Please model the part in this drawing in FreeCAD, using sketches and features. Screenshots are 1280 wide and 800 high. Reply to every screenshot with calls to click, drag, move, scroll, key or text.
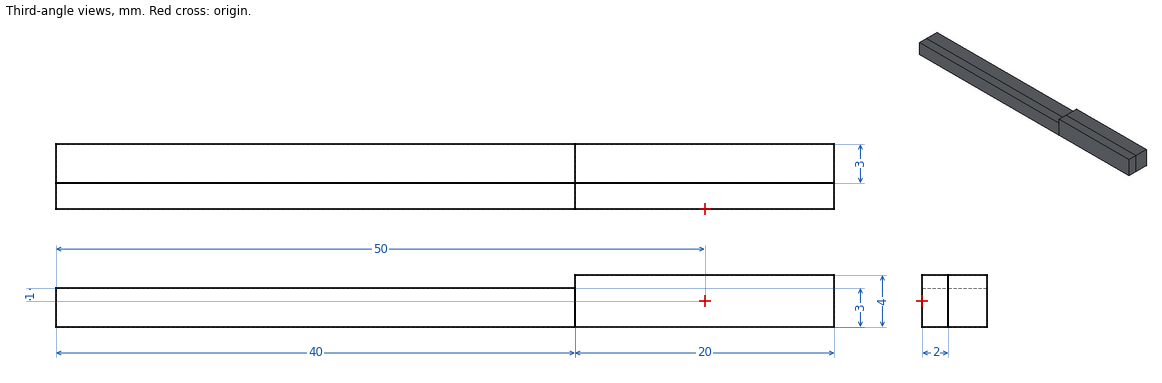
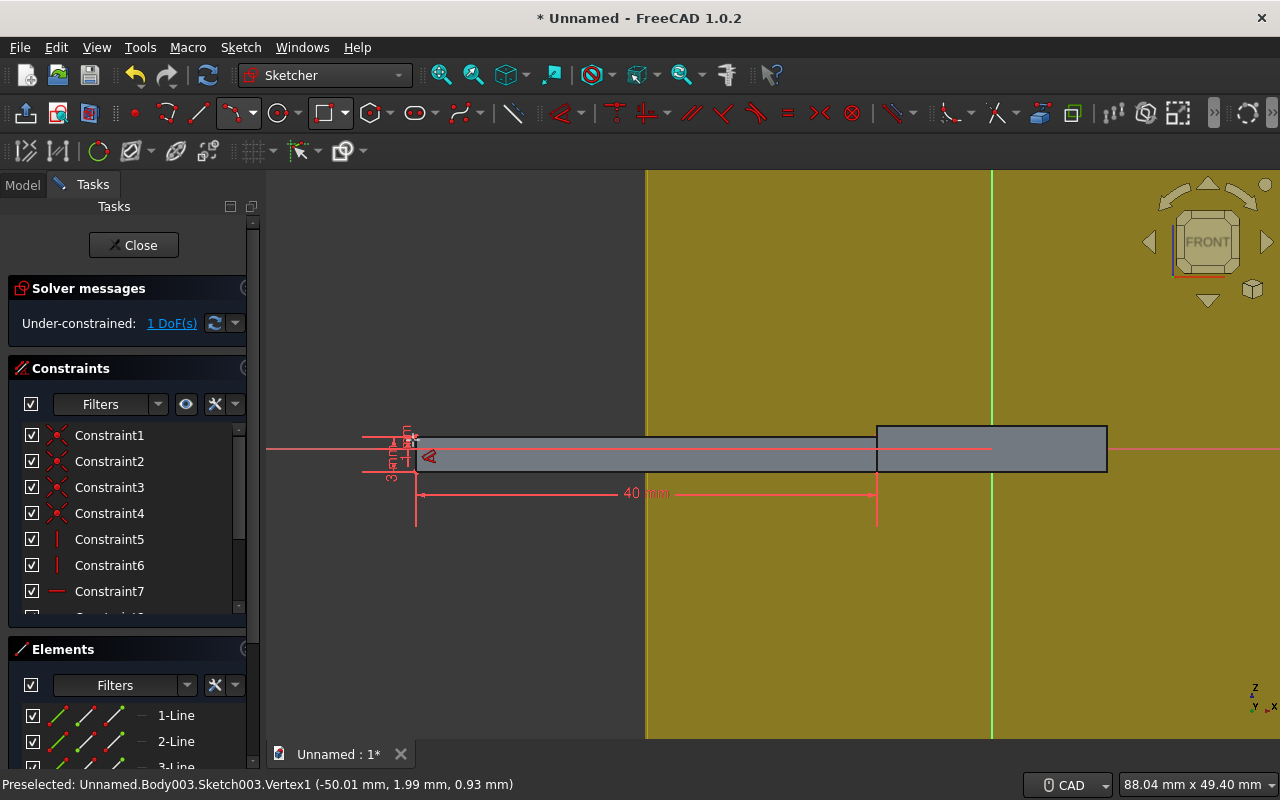
click(416, 437)
click(704, 403)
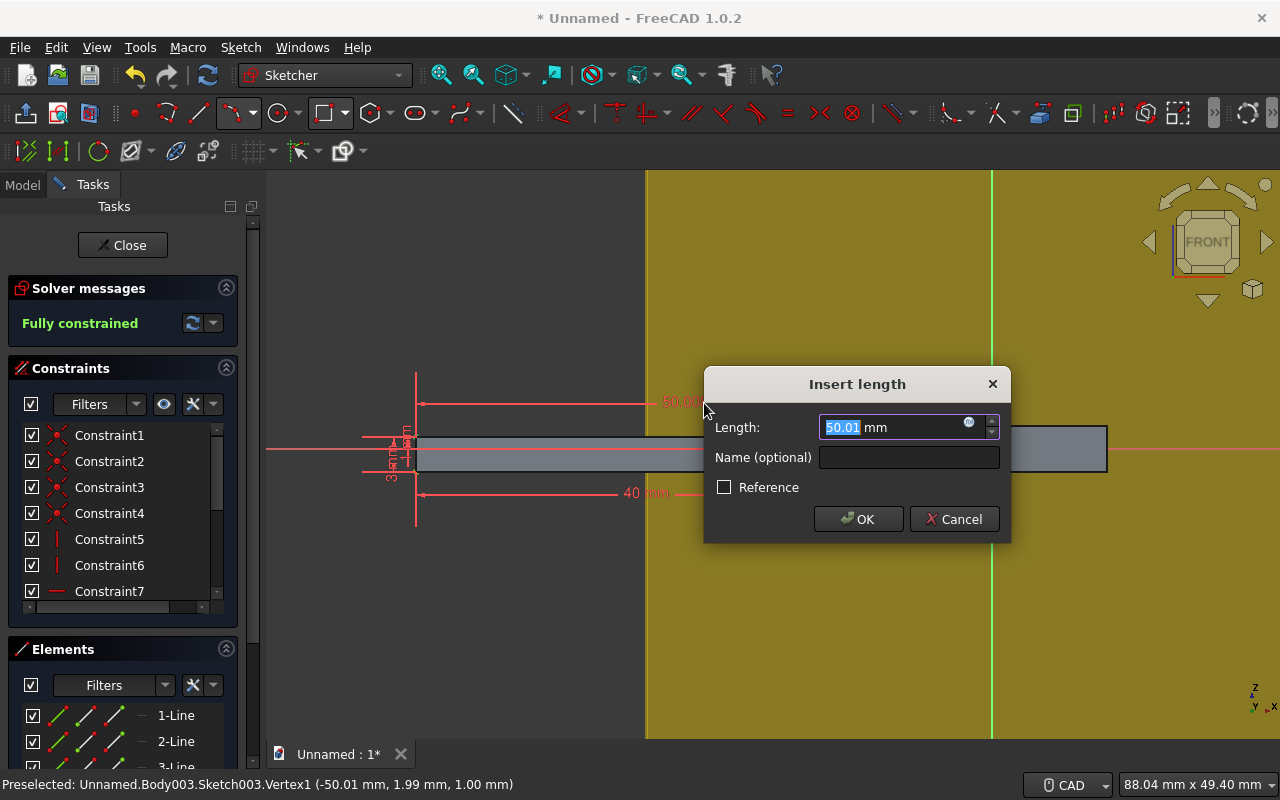
text(50)
key(Return)
key(Escape)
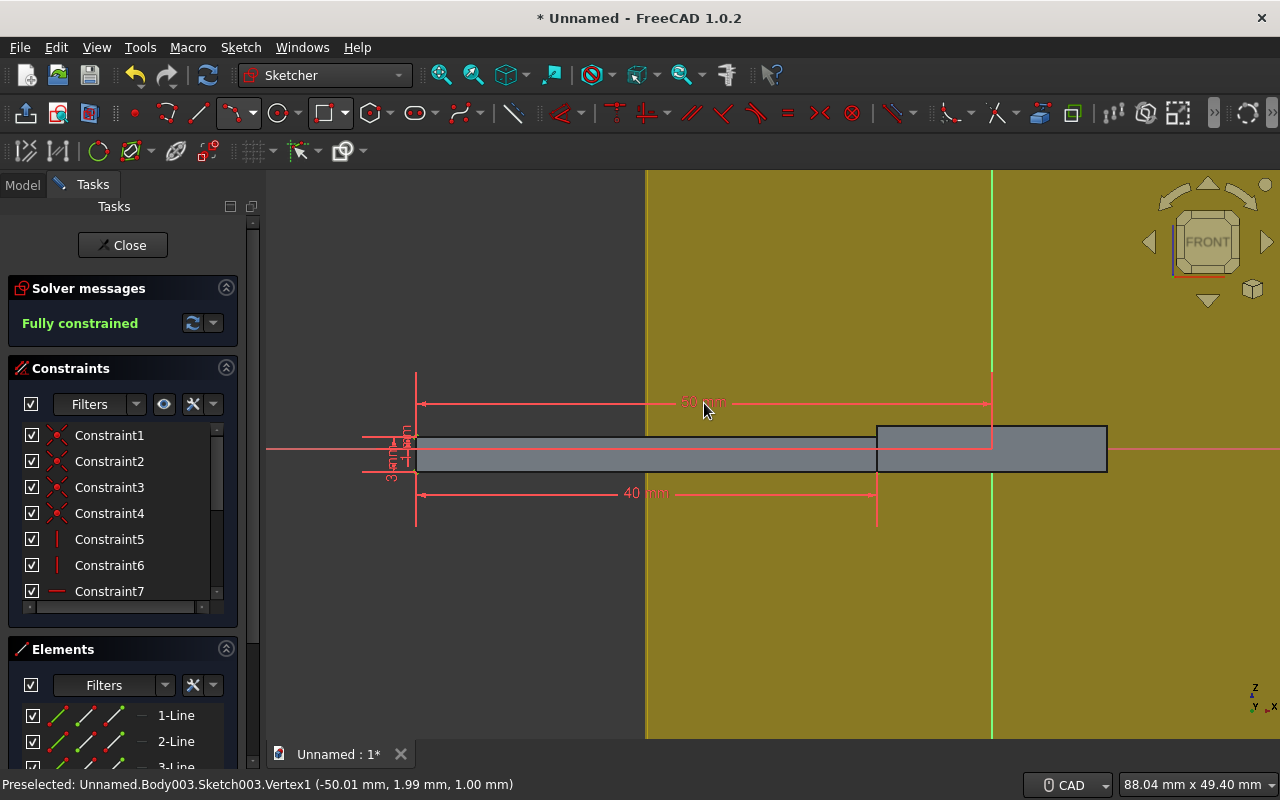
click(123, 245)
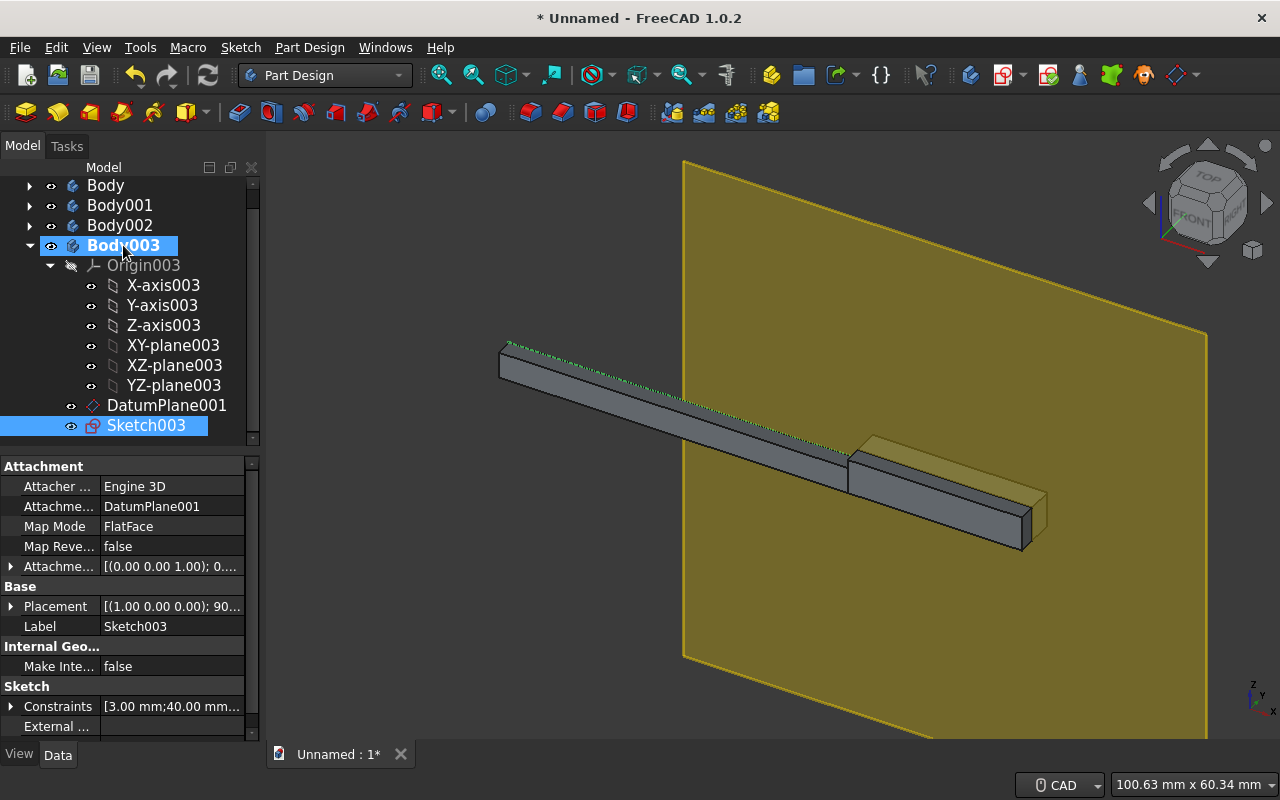
click(26, 112)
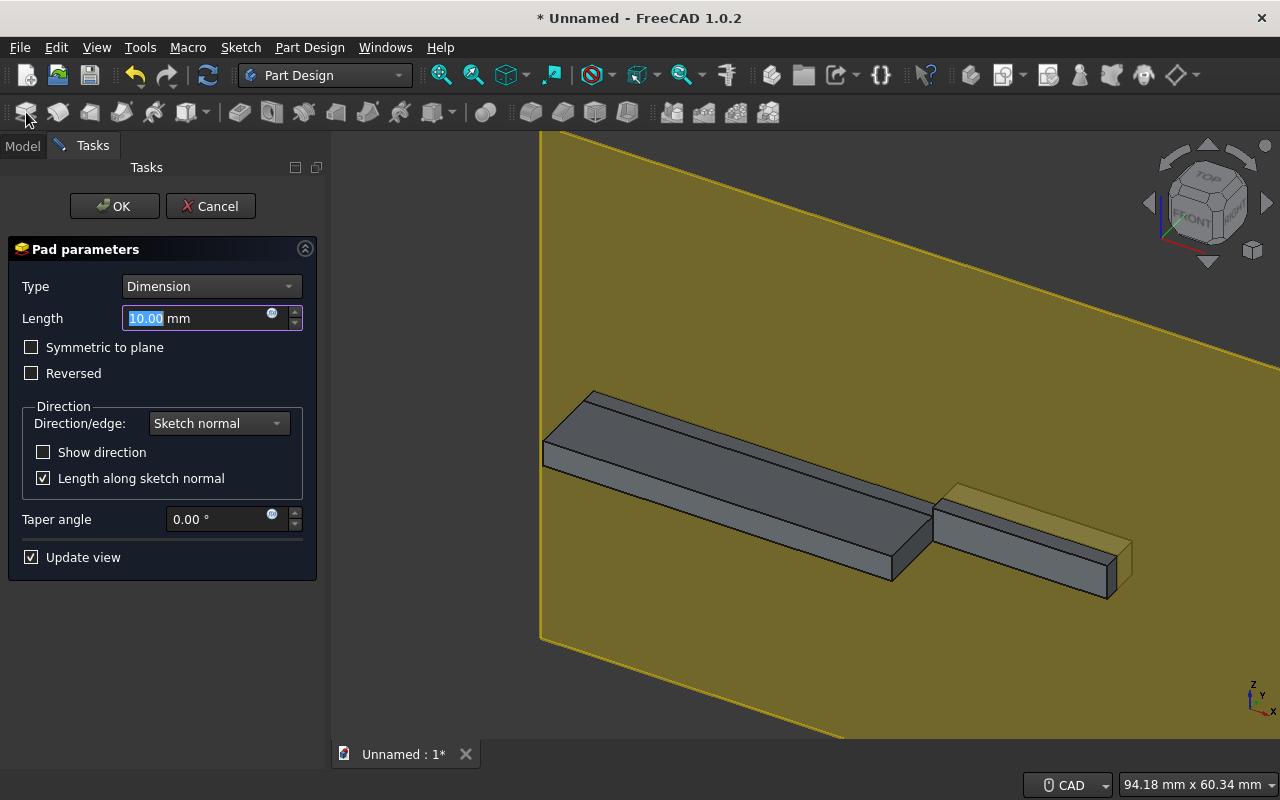
text(3)
key(Tab)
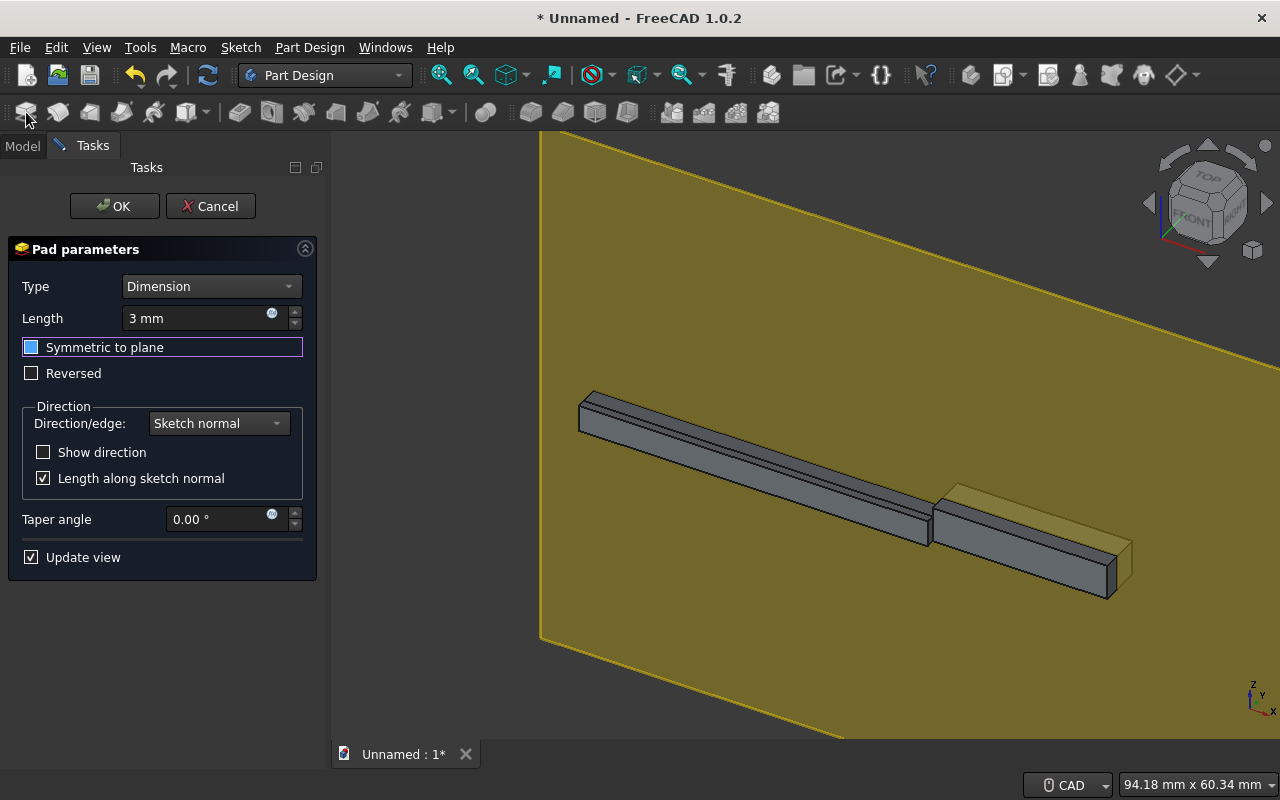
click(30, 373)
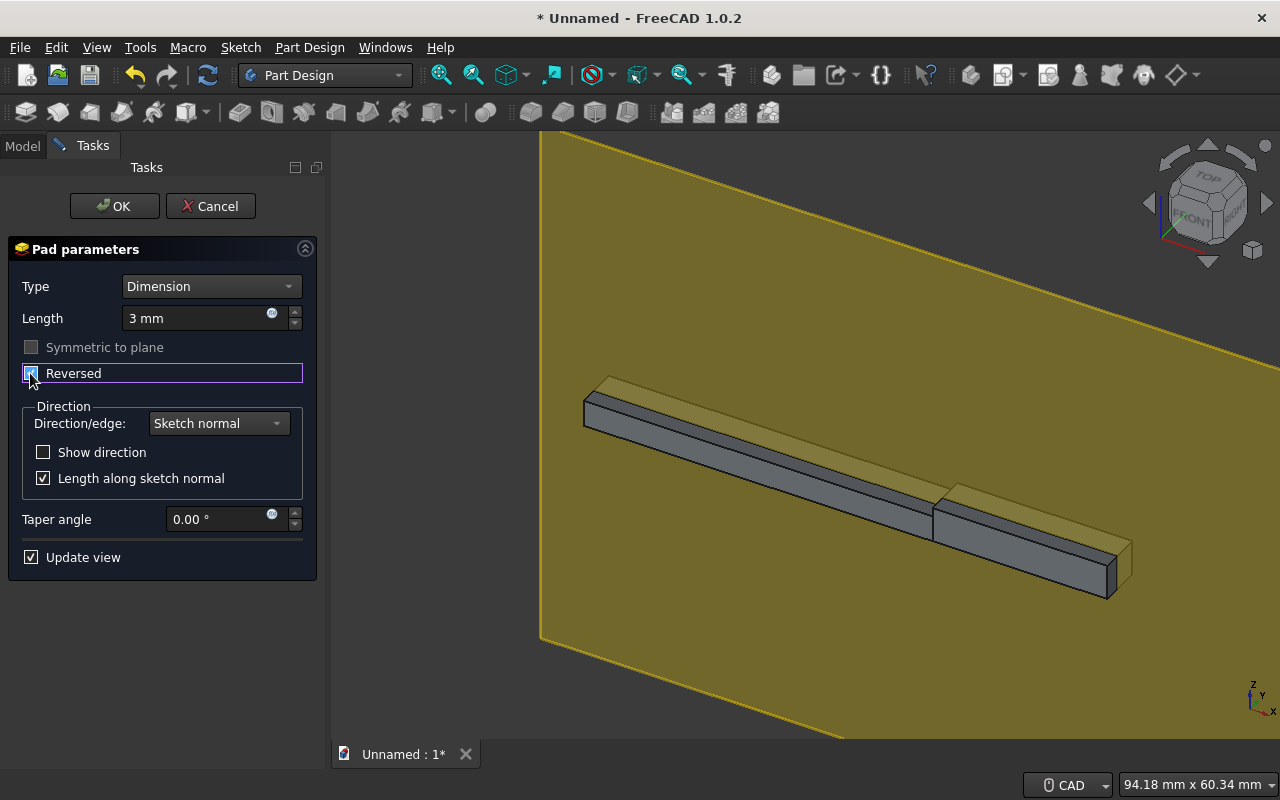
click(115, 206)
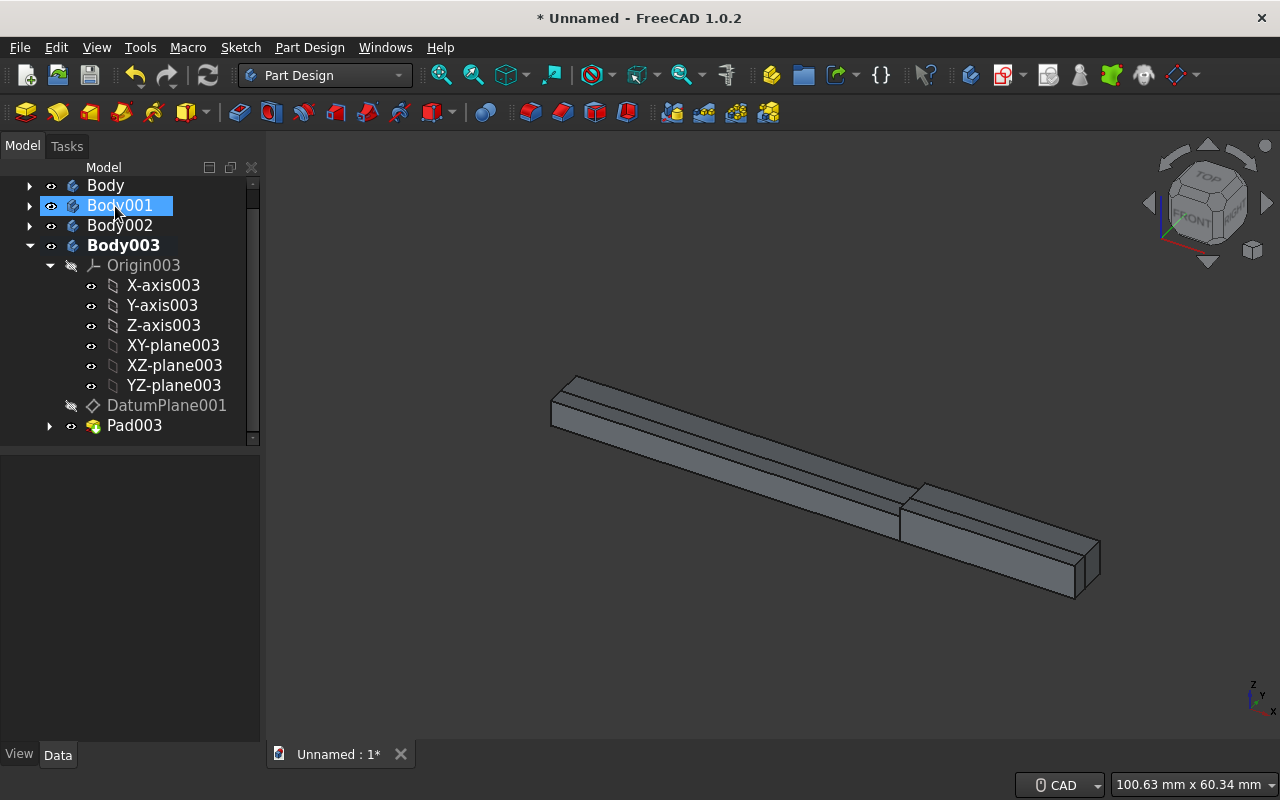
key(0)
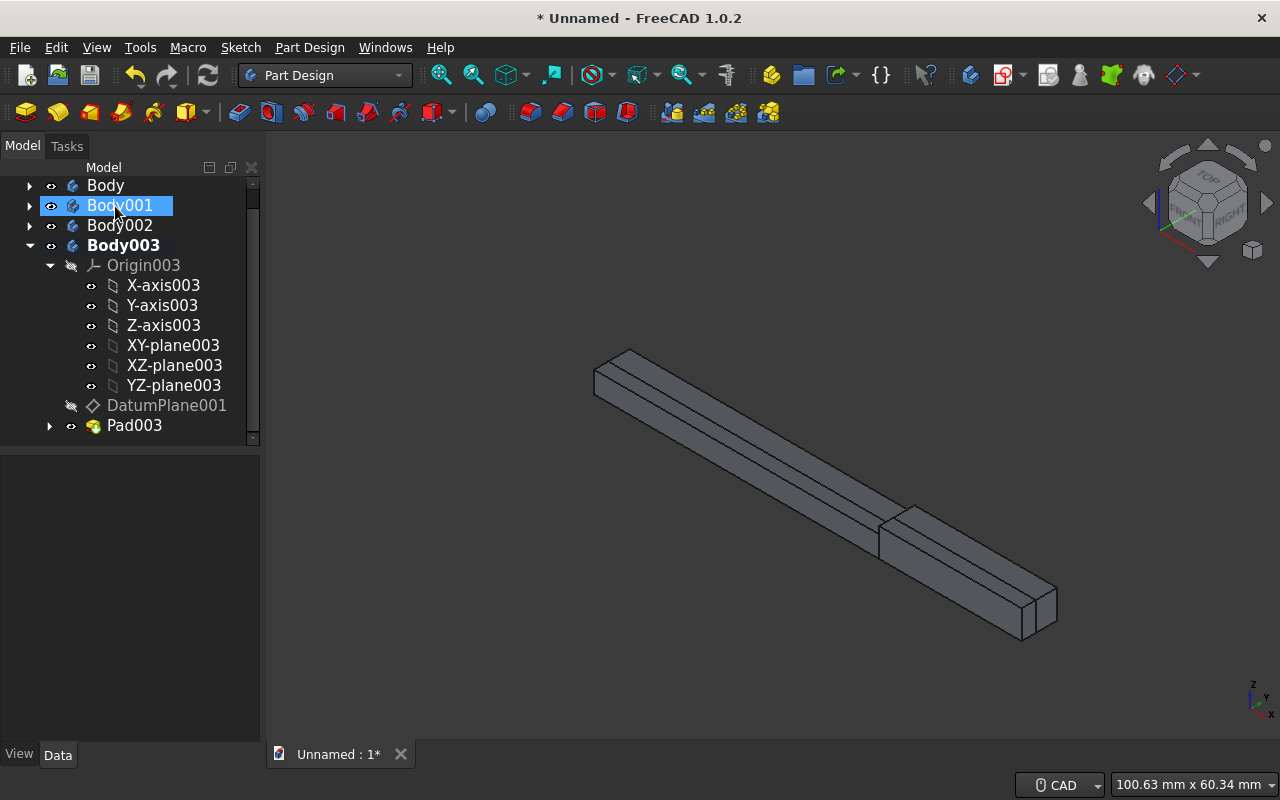
click(442, 76)